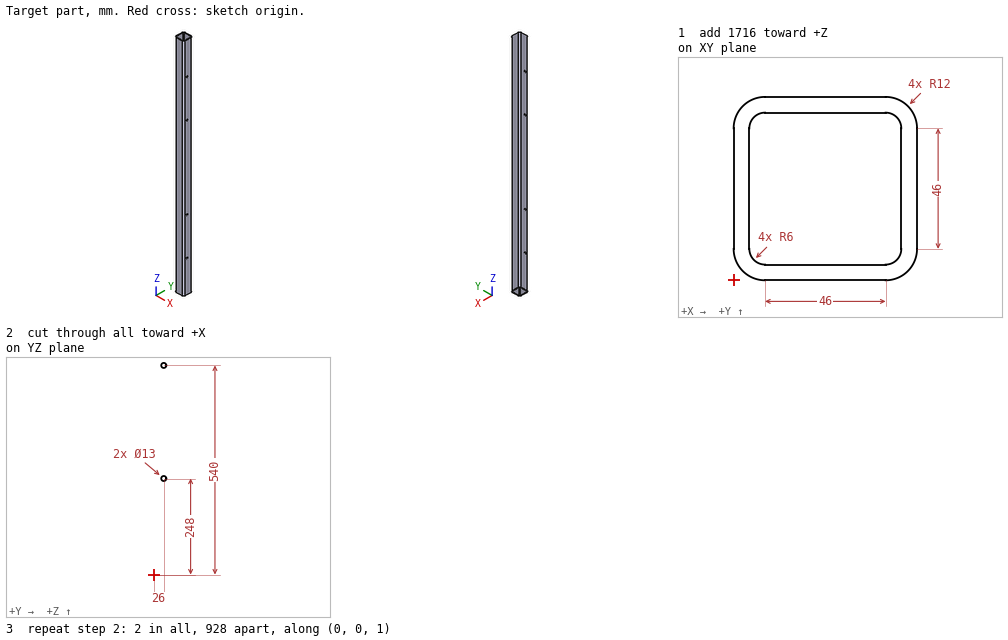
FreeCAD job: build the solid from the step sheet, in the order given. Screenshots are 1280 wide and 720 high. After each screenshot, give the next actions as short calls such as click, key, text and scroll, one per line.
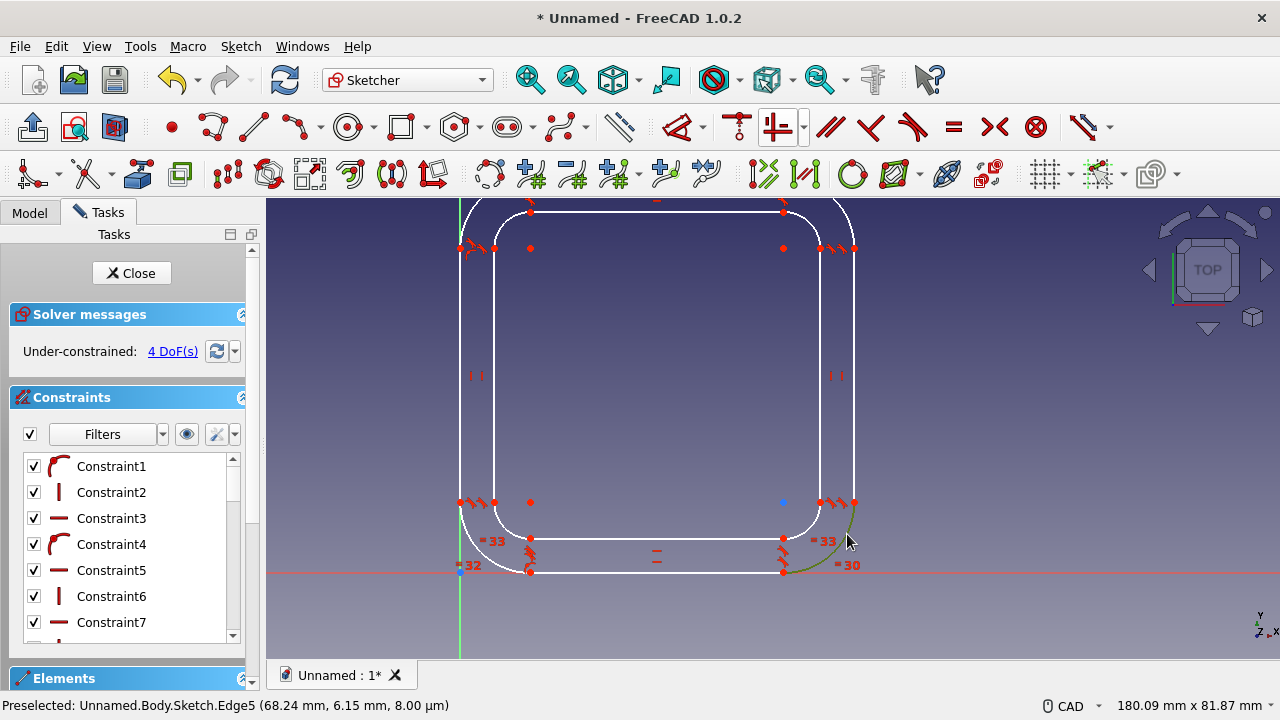
click(702, 128)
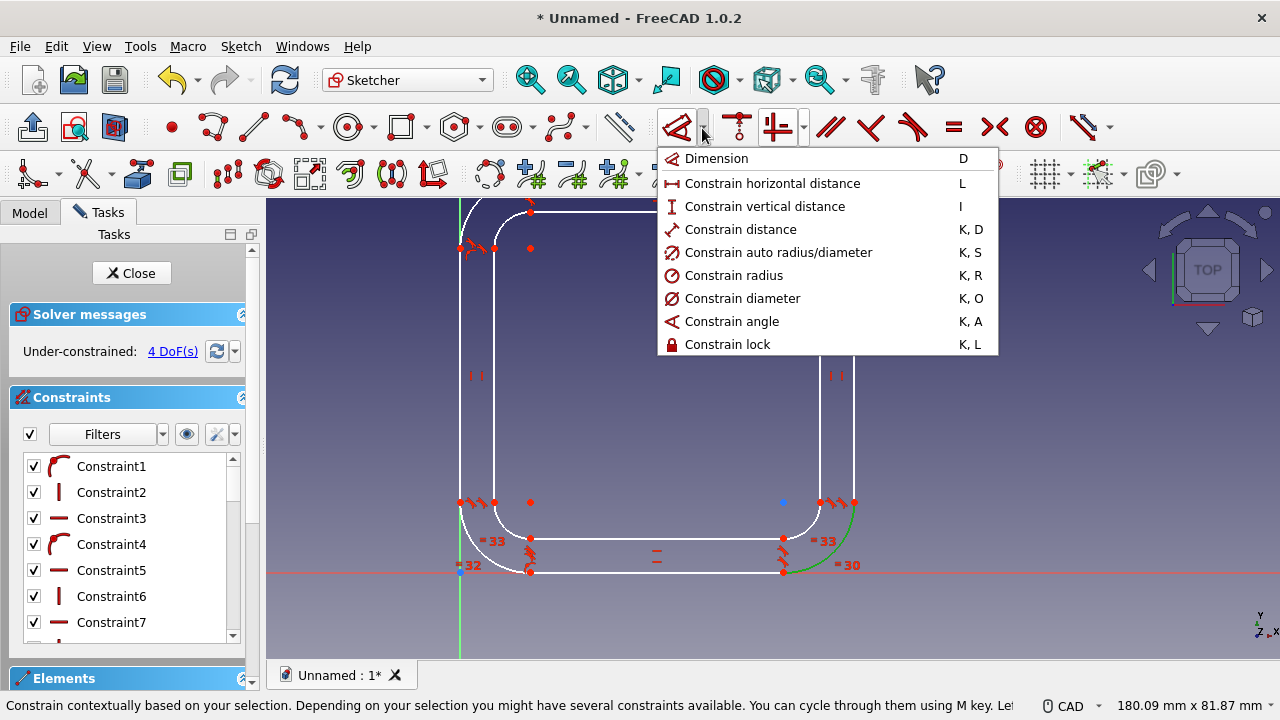
click(828, 276)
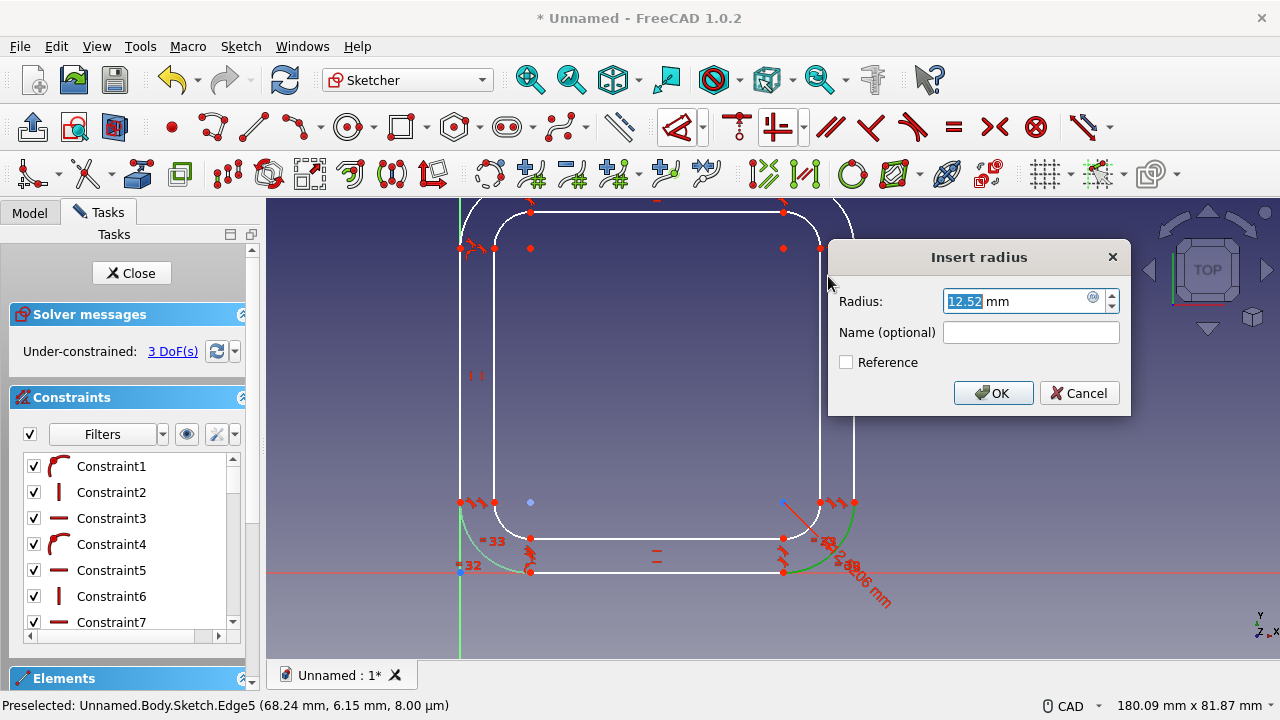
text(12)
key(Return)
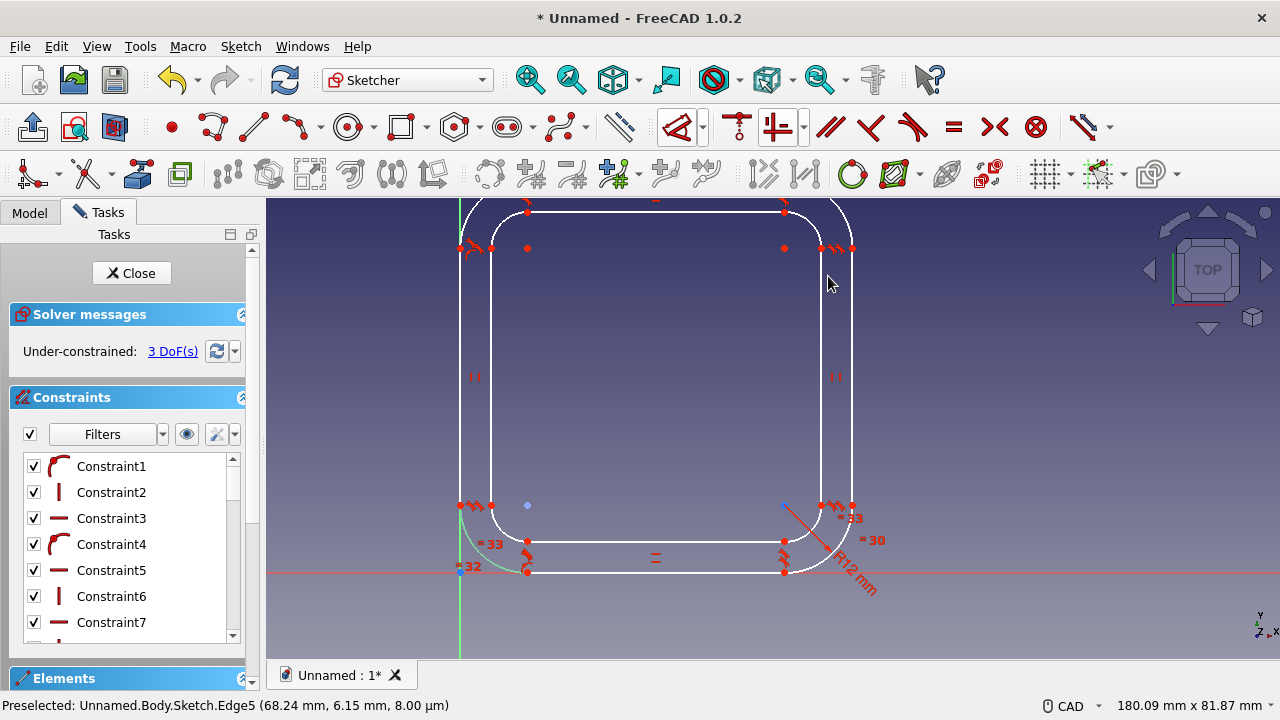
click(495, 522)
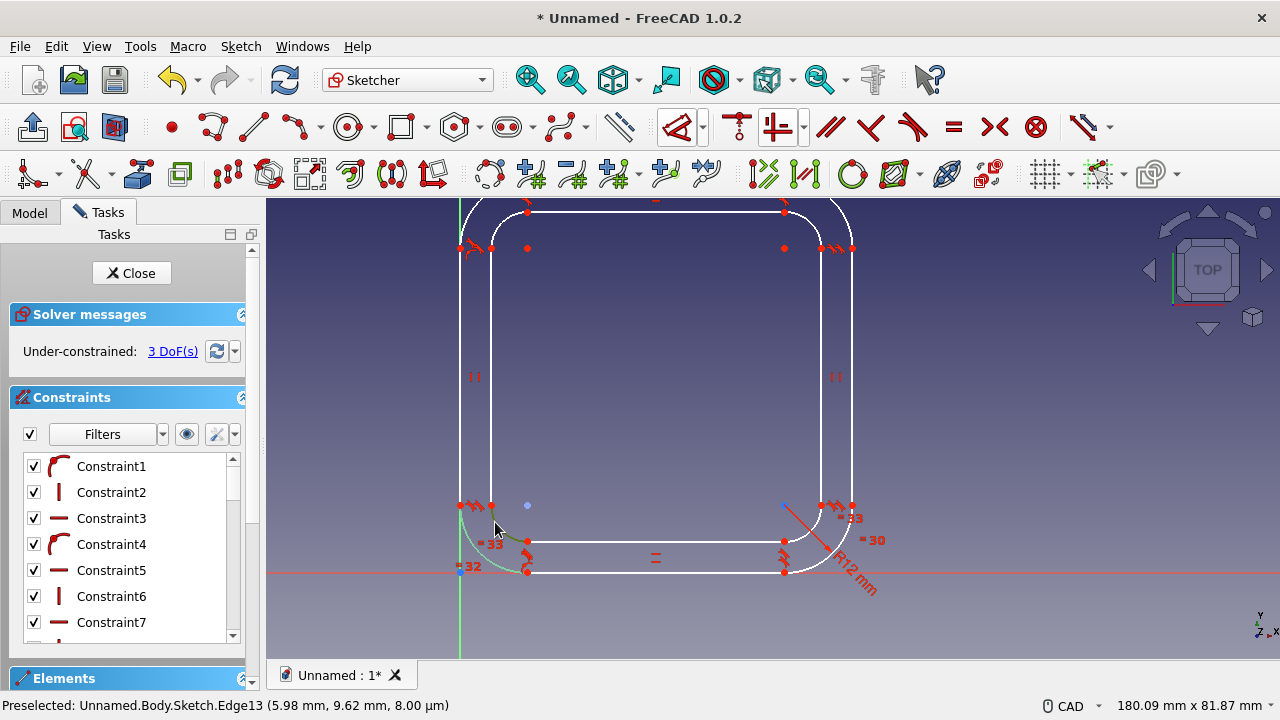
click(702, 128)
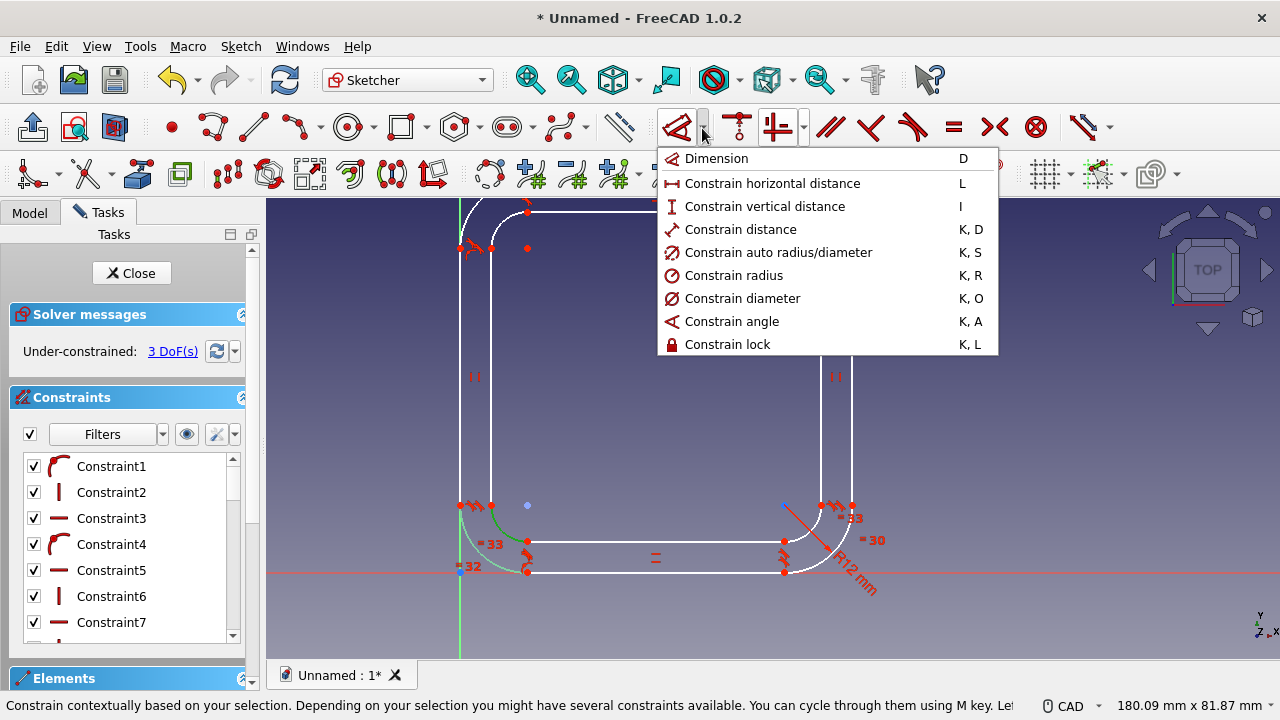
click(828, 276)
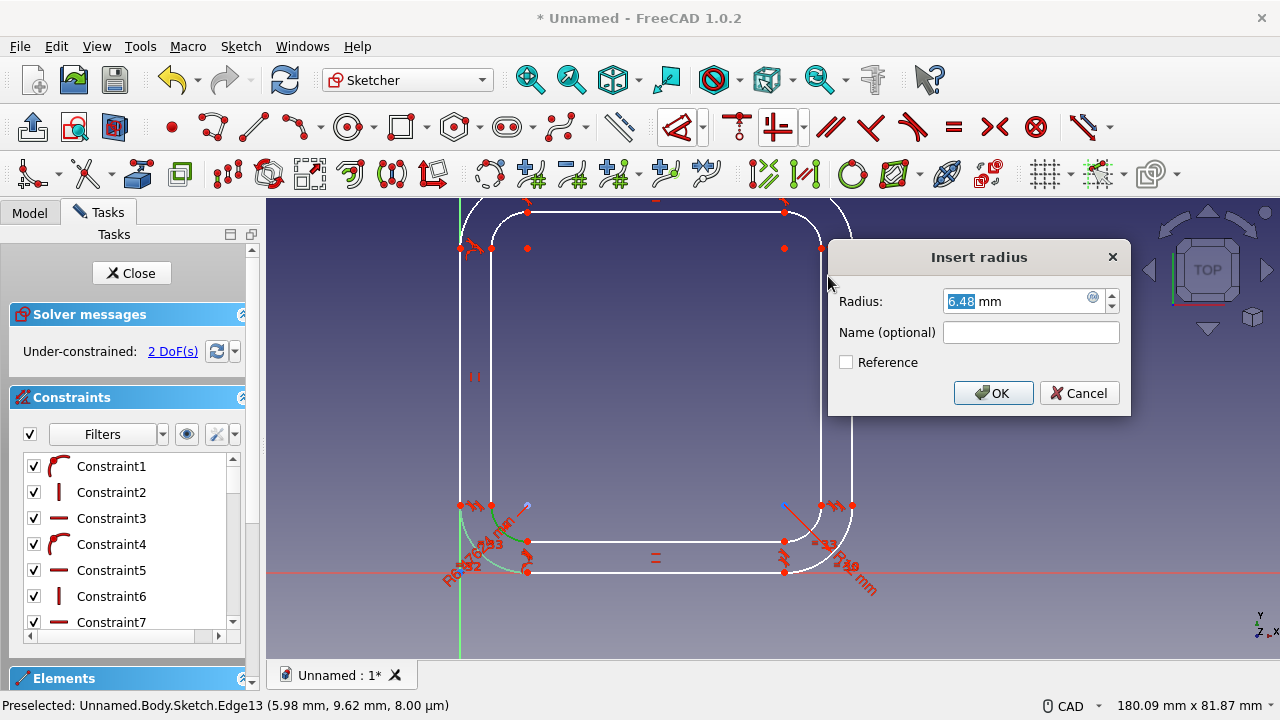
text(6)
key(Return)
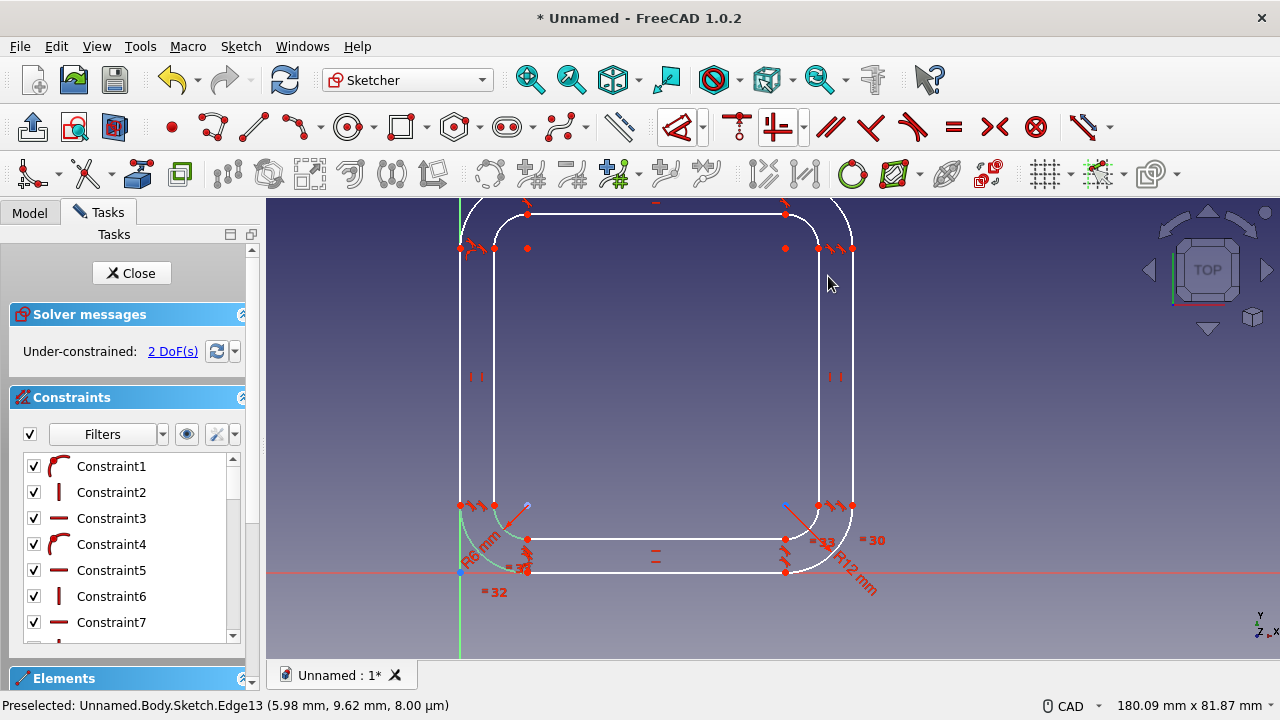
click(605, 573)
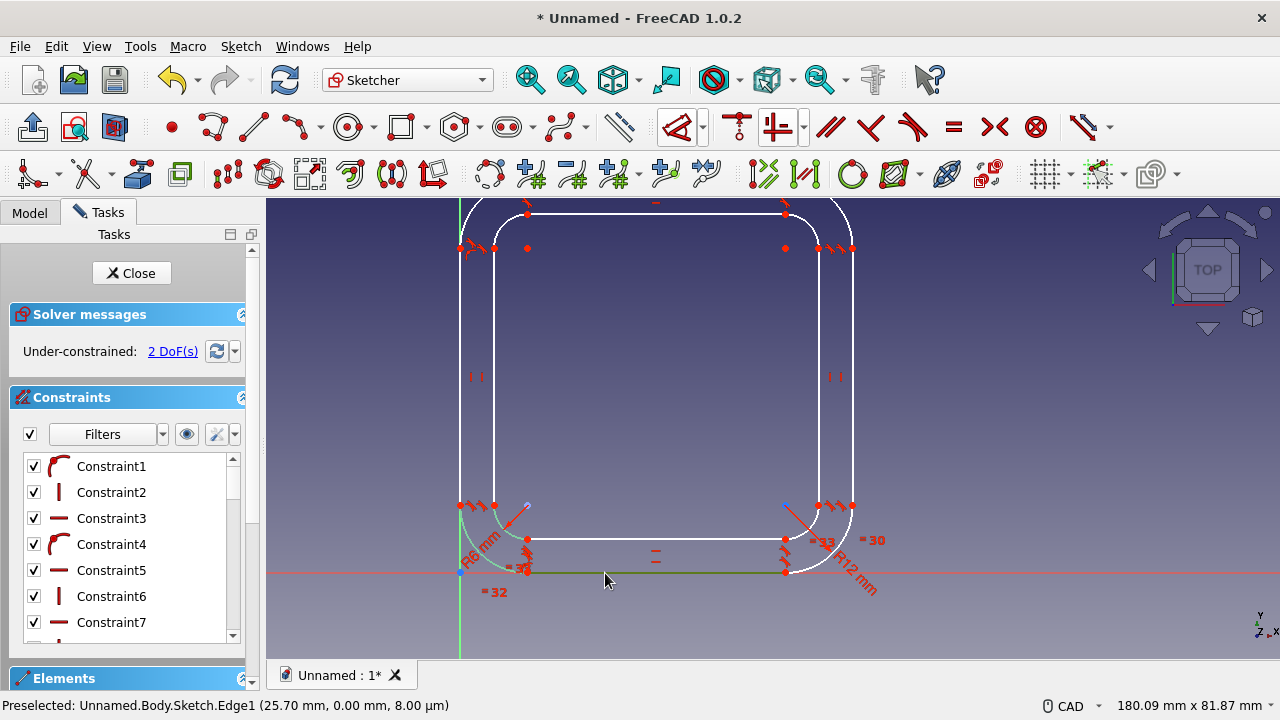
click(702, 128)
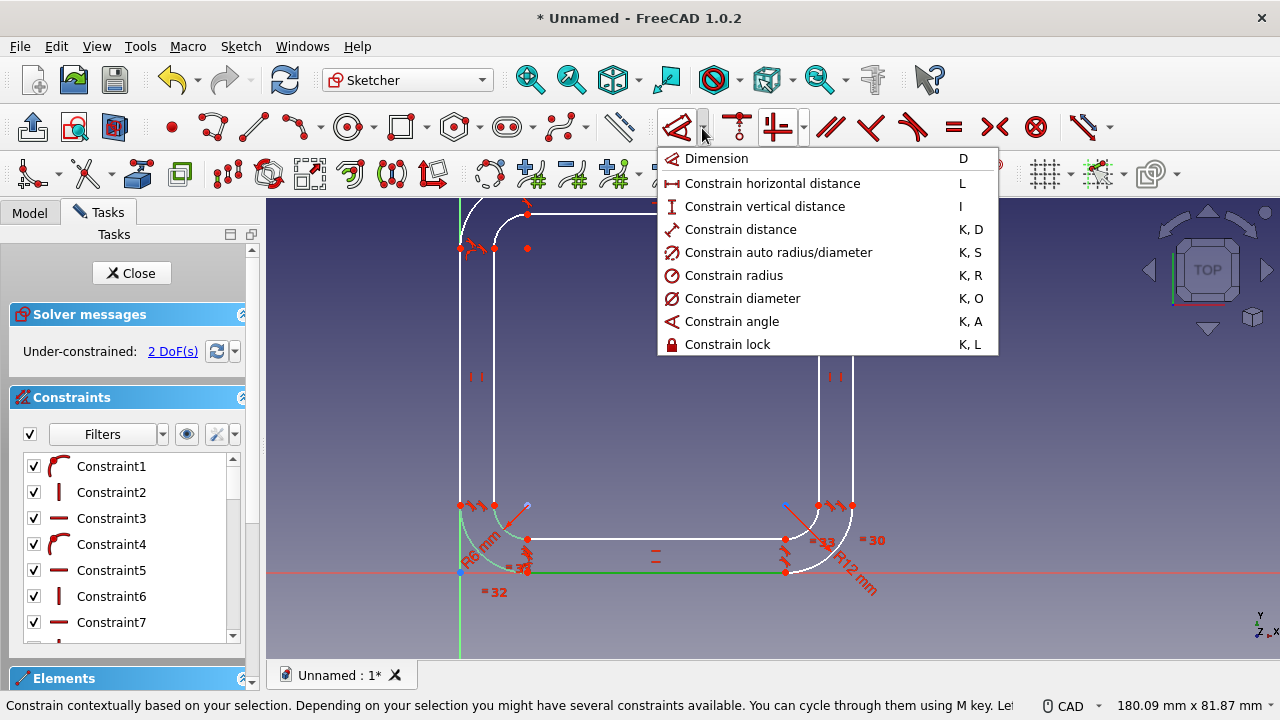
click(828, 184)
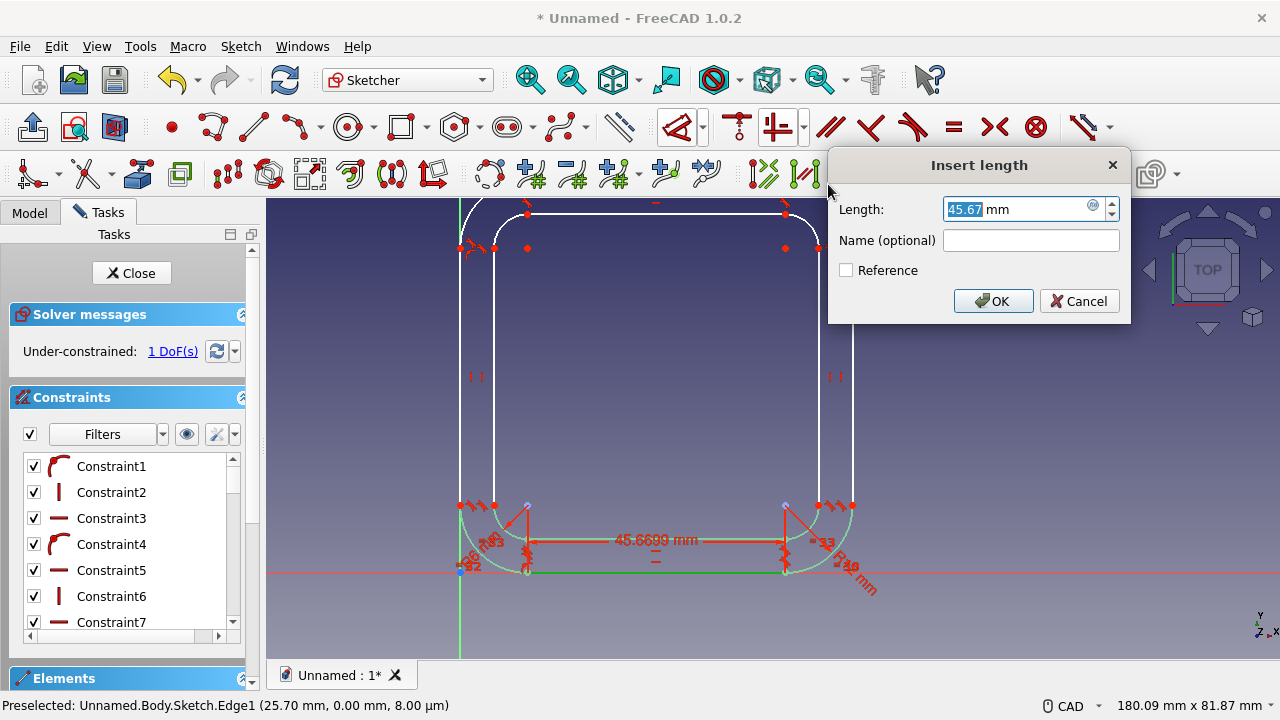
text(46)
key(Return)